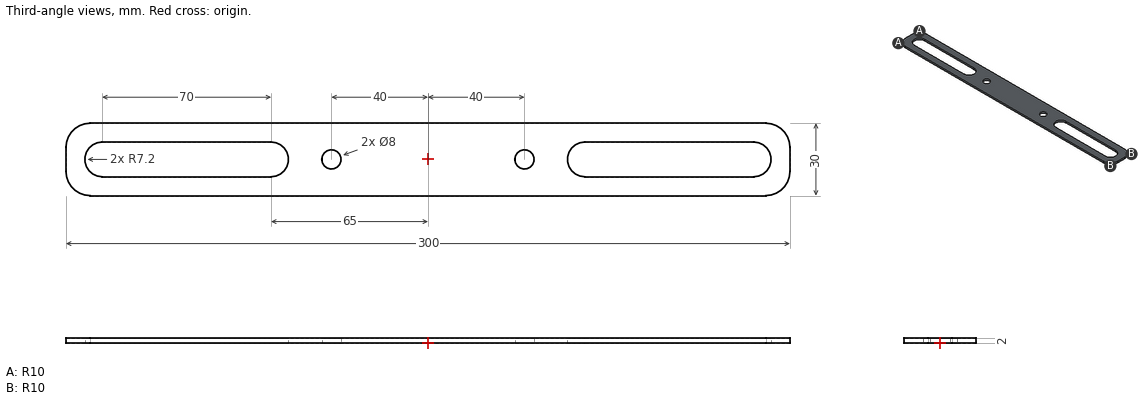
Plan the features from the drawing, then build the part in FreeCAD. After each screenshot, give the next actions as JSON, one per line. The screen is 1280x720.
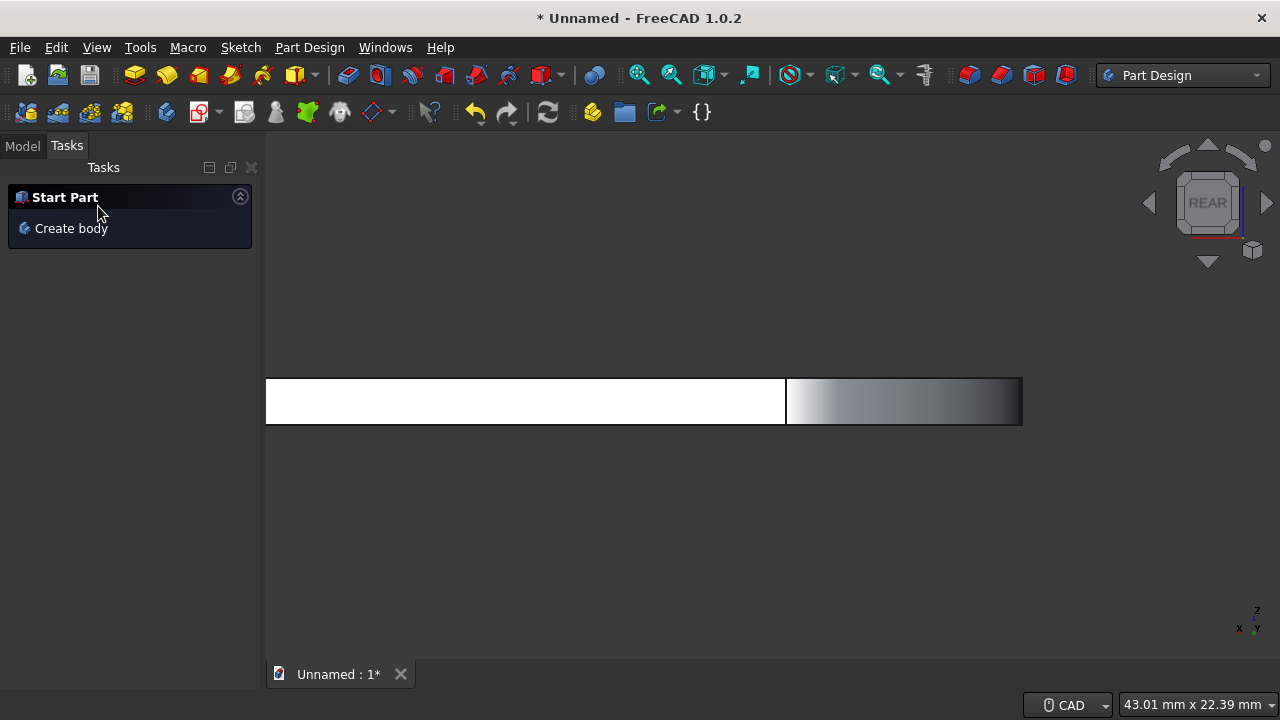
{"action": "left_click", "coordinate": [640, 76]}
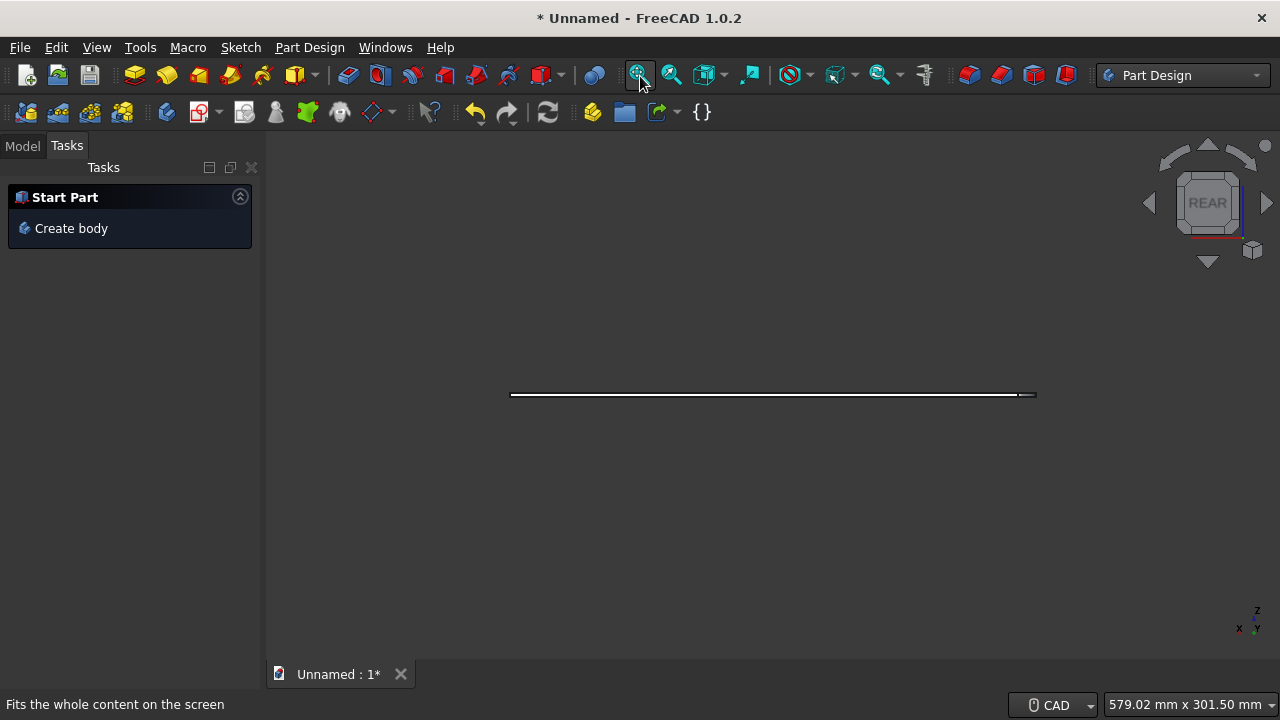
{"action": "left_click", "coordinate": [23, 145]}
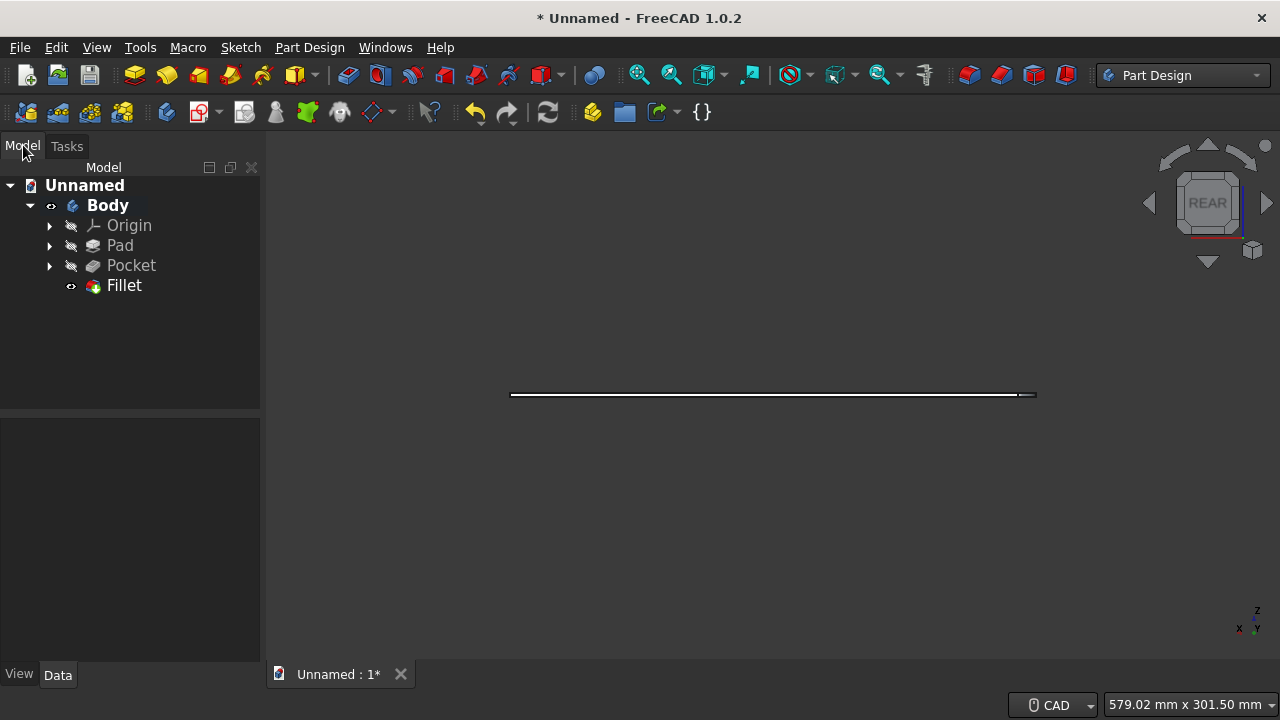
{"action": "left_click", "coordinate": [116, 266]}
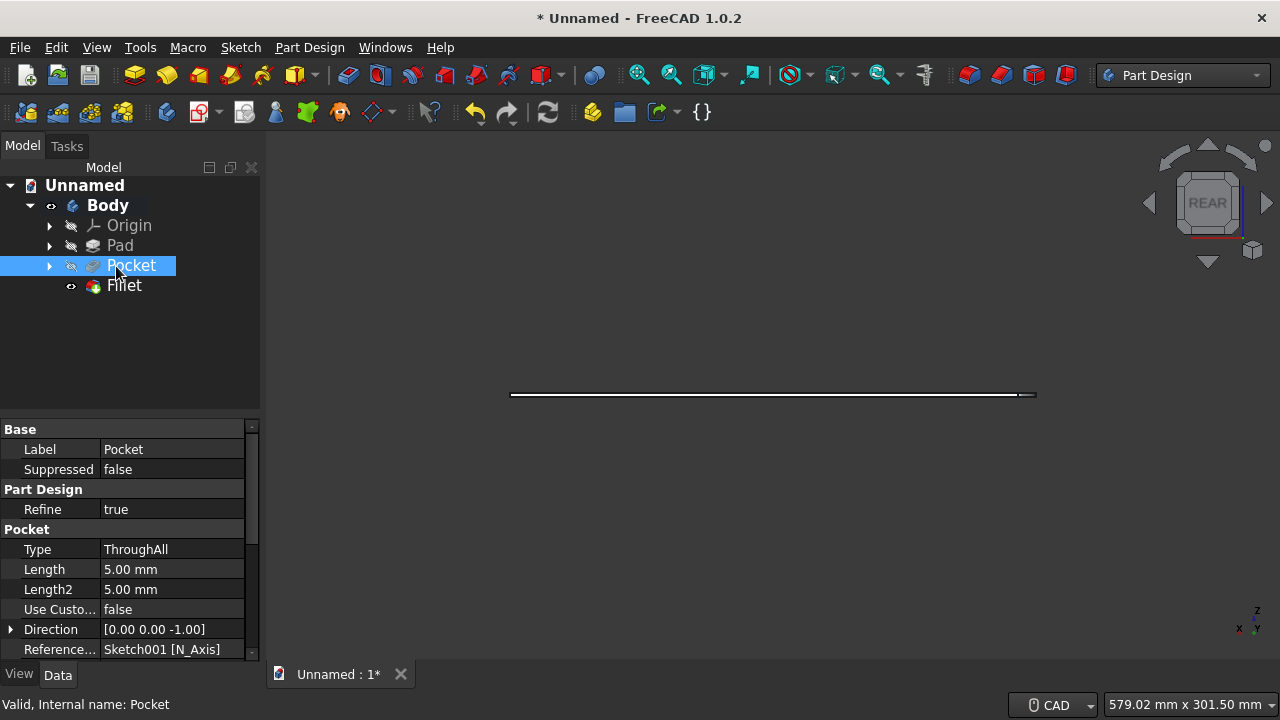
{"action": "left_click", "coordinate": [26, 112]}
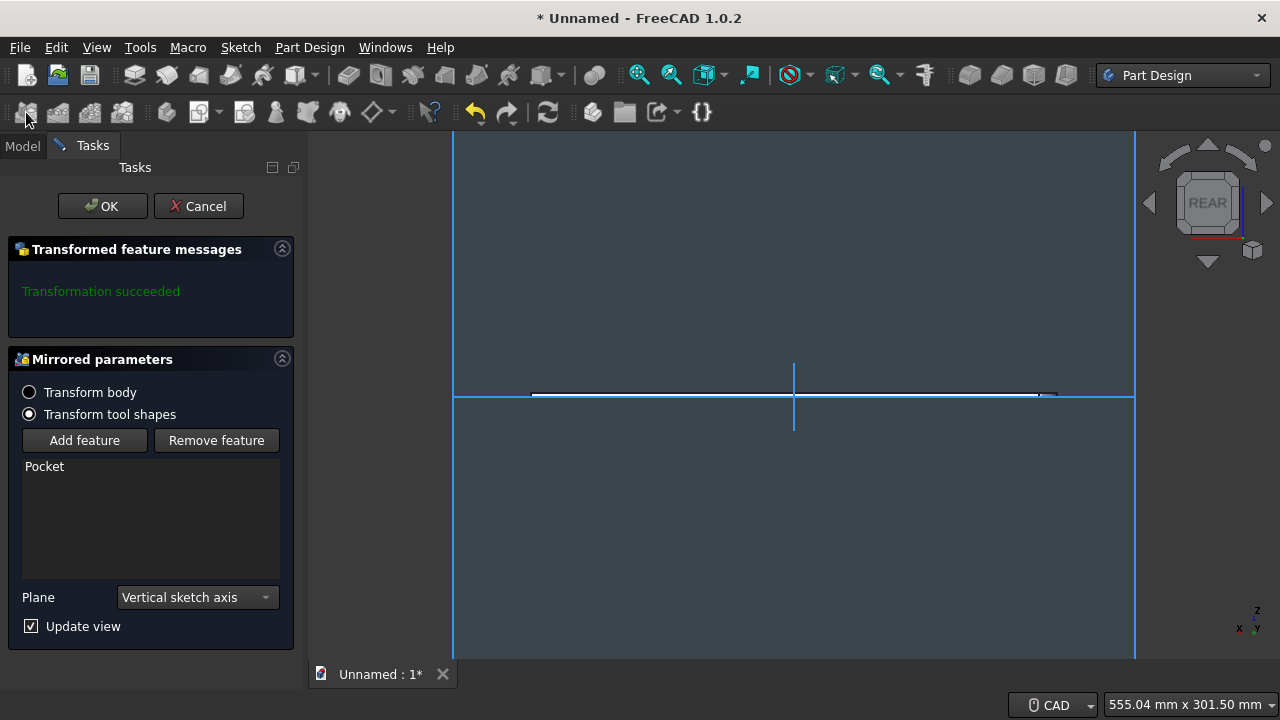
{"action": "left_click", "coordinate": [198, 598]}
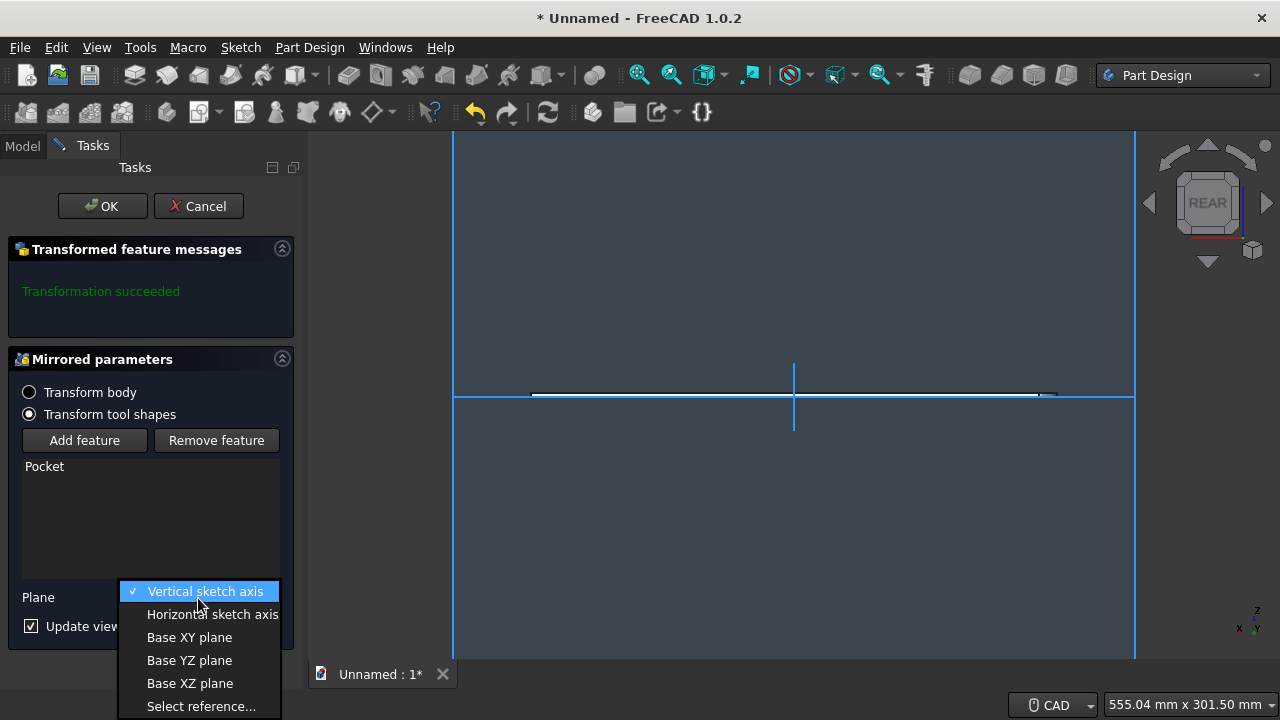
{"action": "left_click", "coordinate": [198, 660]}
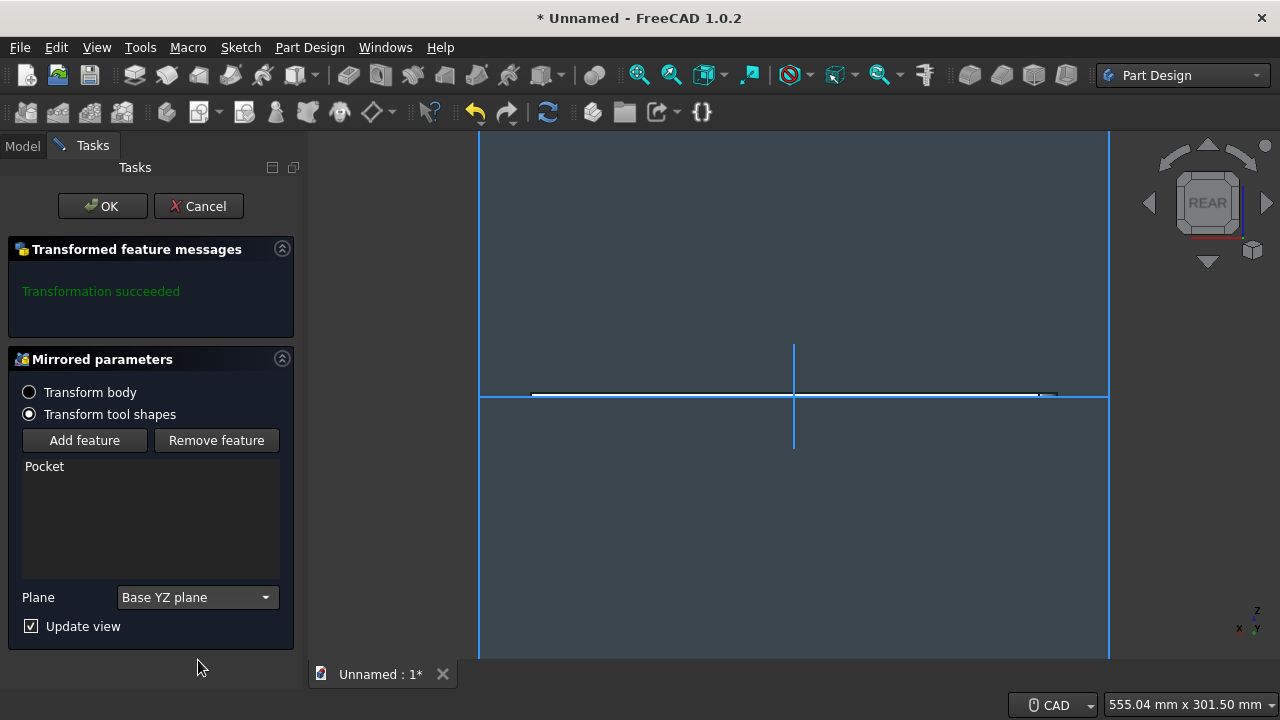
{"action": "left_click", "coordinate": [103, 206]}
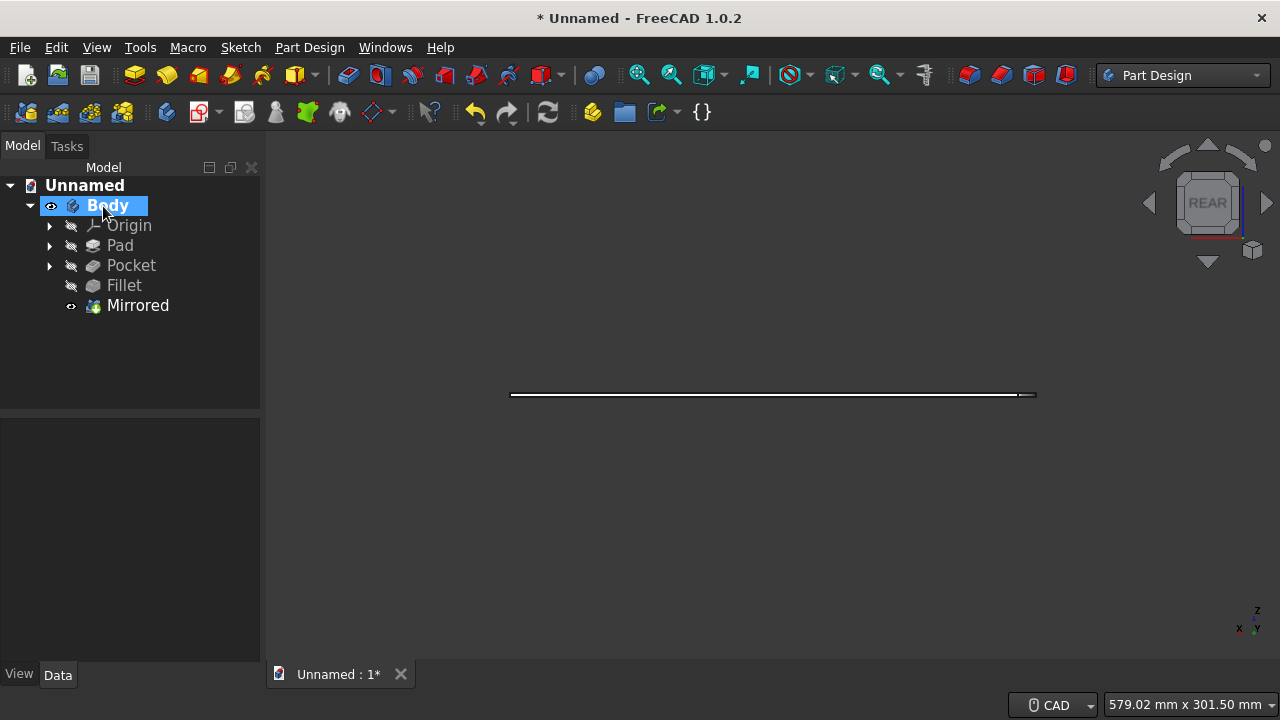
{"action": "scroll", "coordinate": [510, 394], "scroll_direction": "up", "scroll_amount": 13}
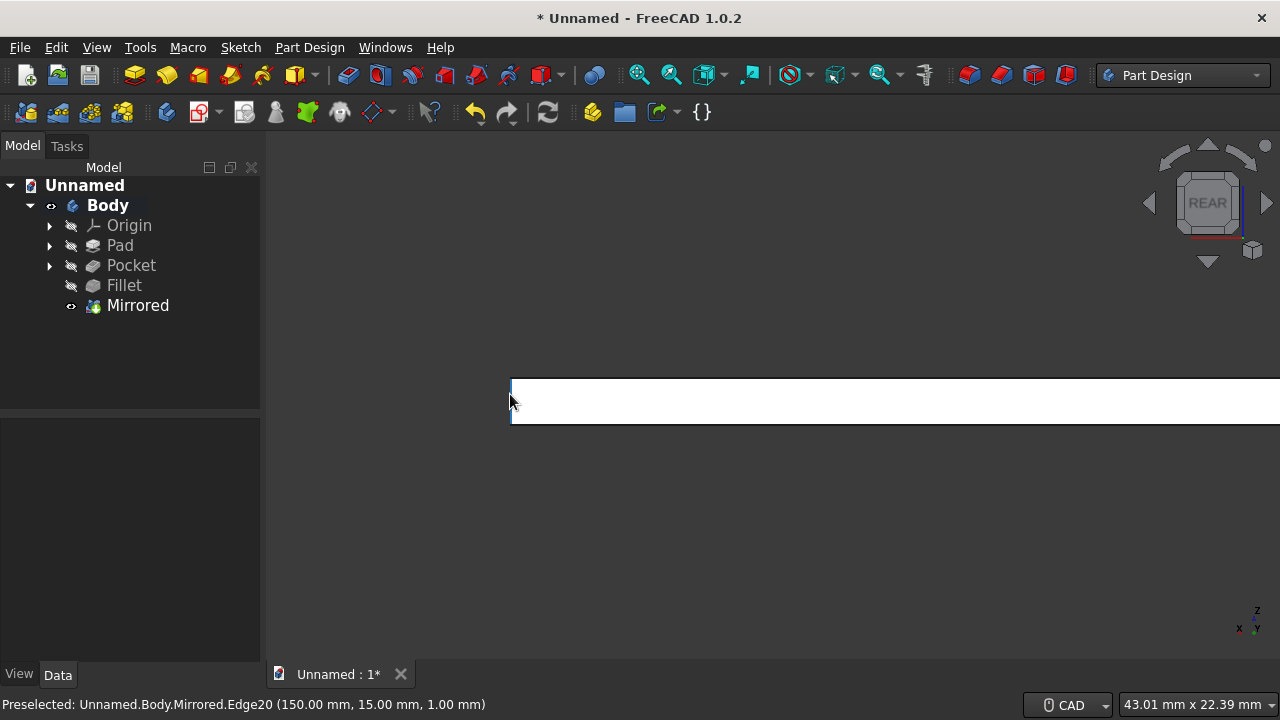
{"action": "left_click", "coordinate": [511, 400]}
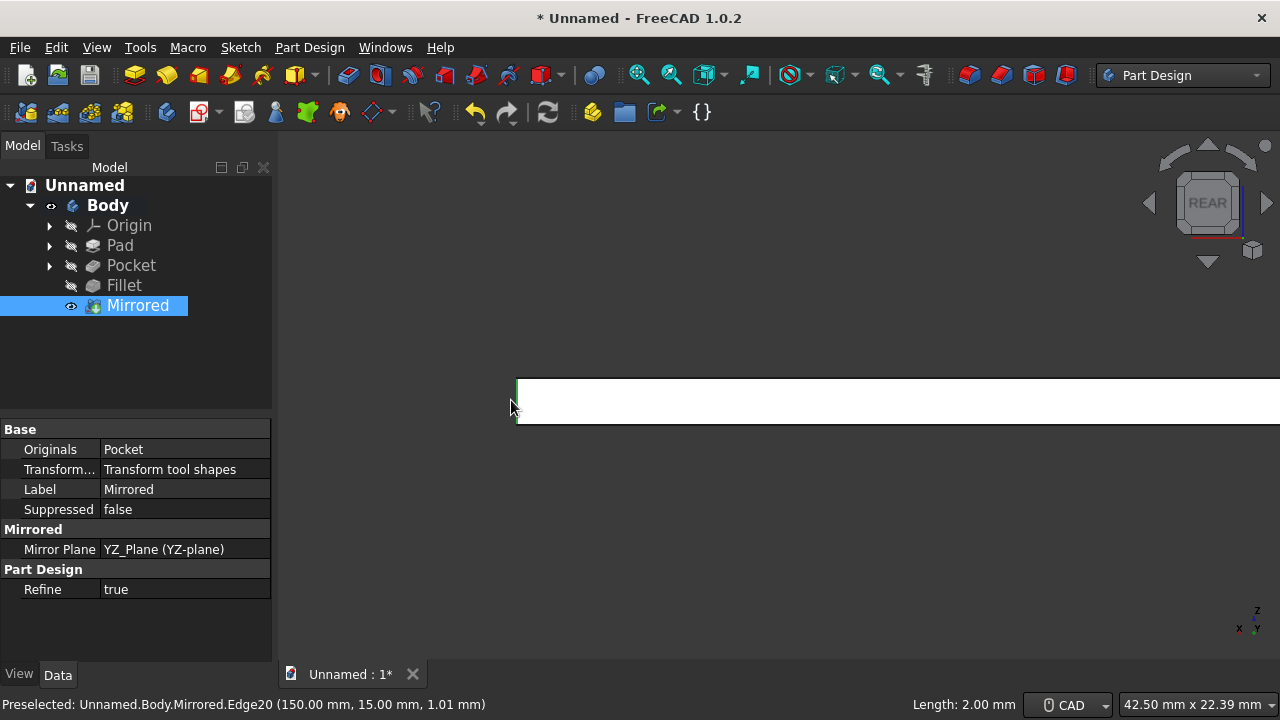
{"action": "key", "text": "v f"}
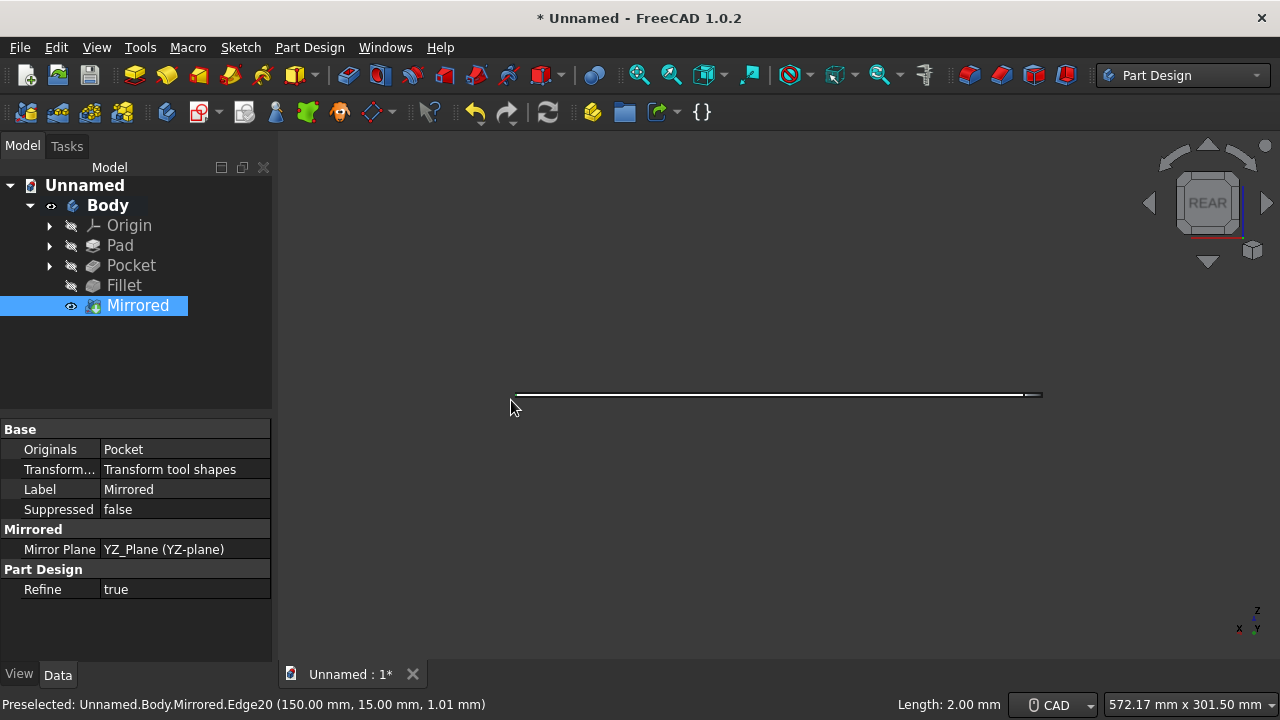
{"action": "key", "text": "0"}